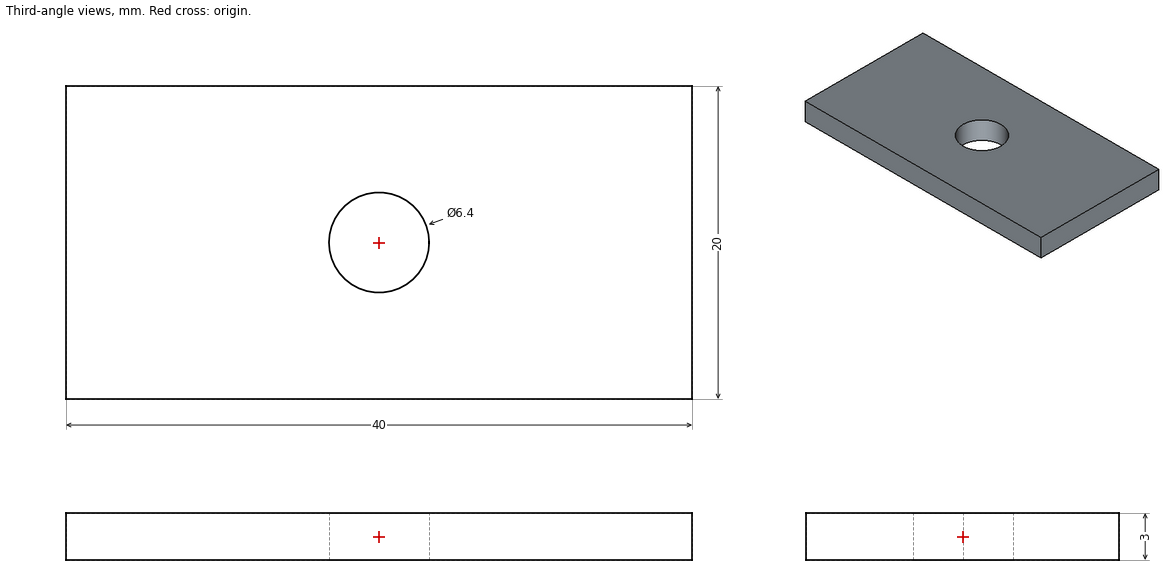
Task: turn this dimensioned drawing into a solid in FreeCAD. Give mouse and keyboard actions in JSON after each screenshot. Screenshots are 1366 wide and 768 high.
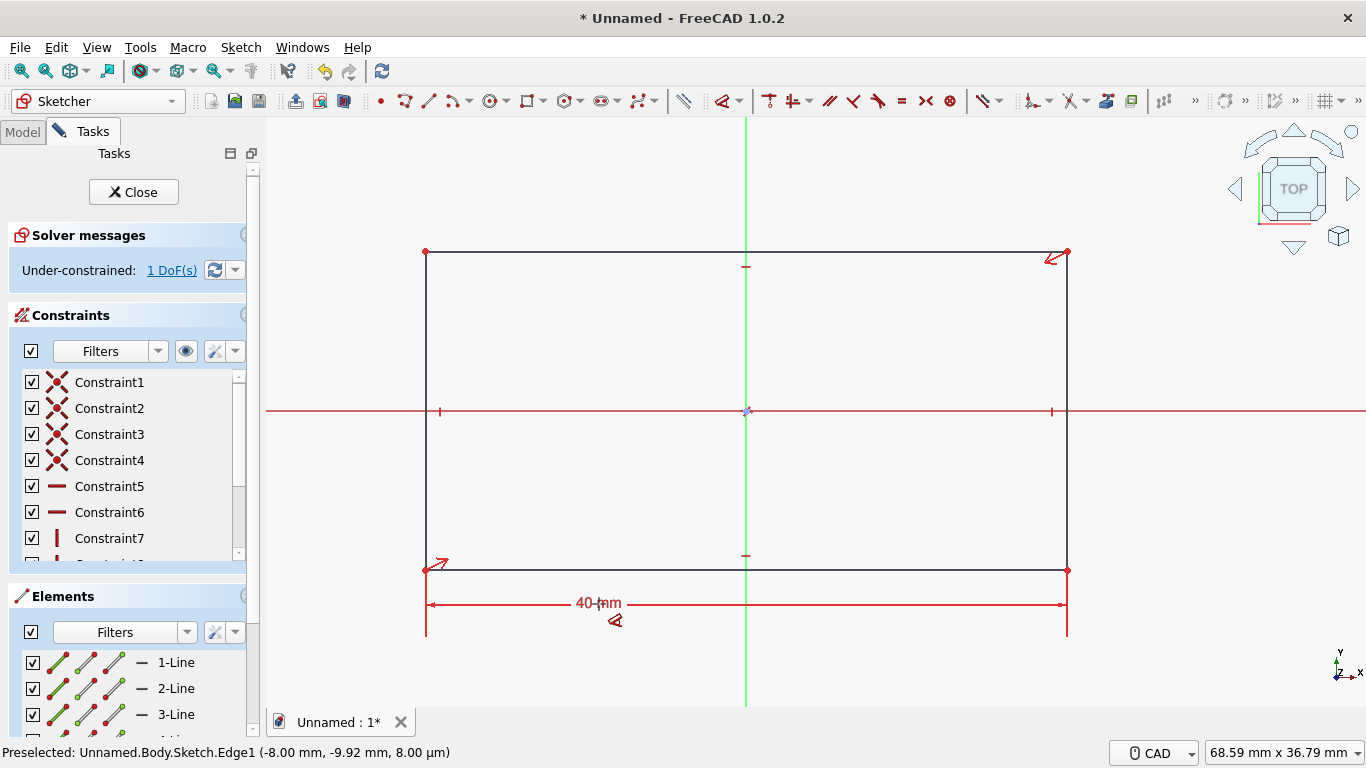
{"action": "left_click", "coordinate": [1067, 475]}
{"action": "left_click", "coordinate": [1101, 338]}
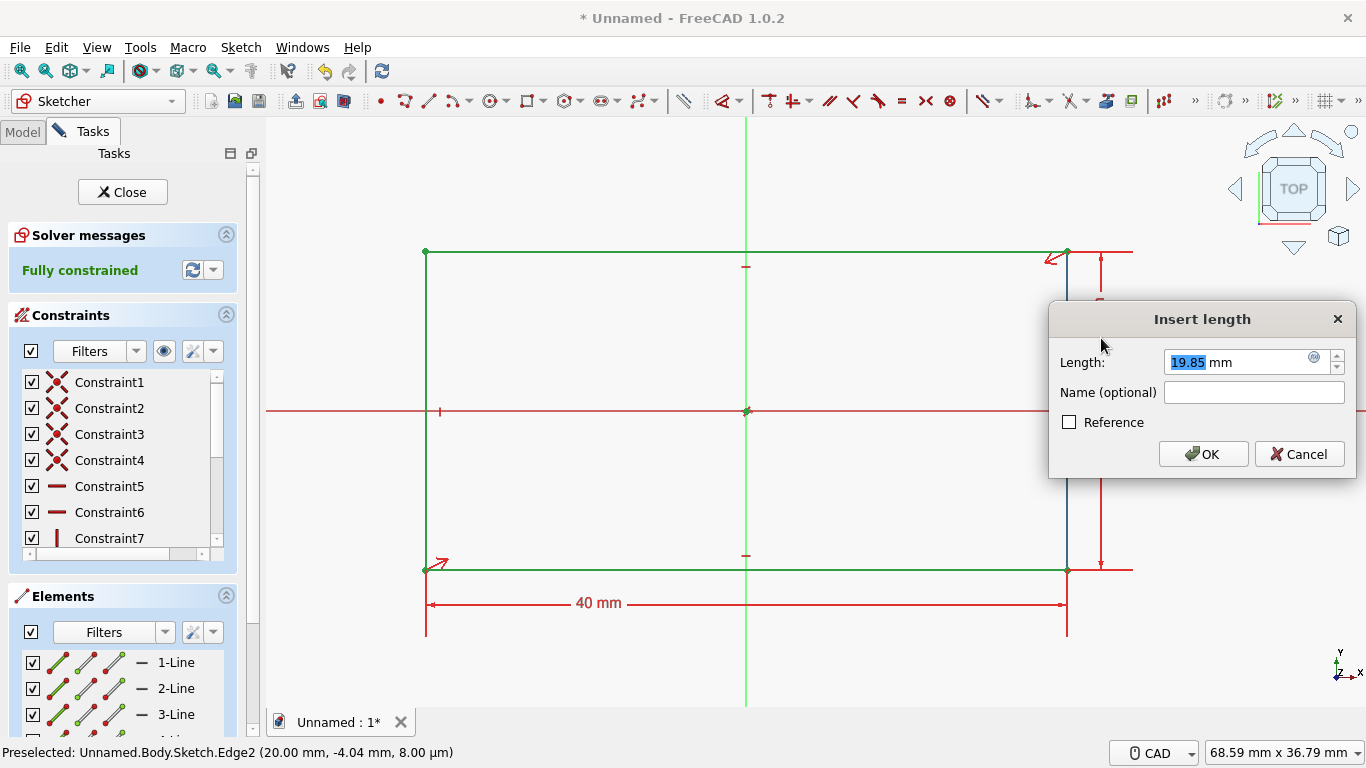
{"action": "type", "text": "20"}
{"action": "key", "text": "Return"}
{"action": "key", "text": "Escape"}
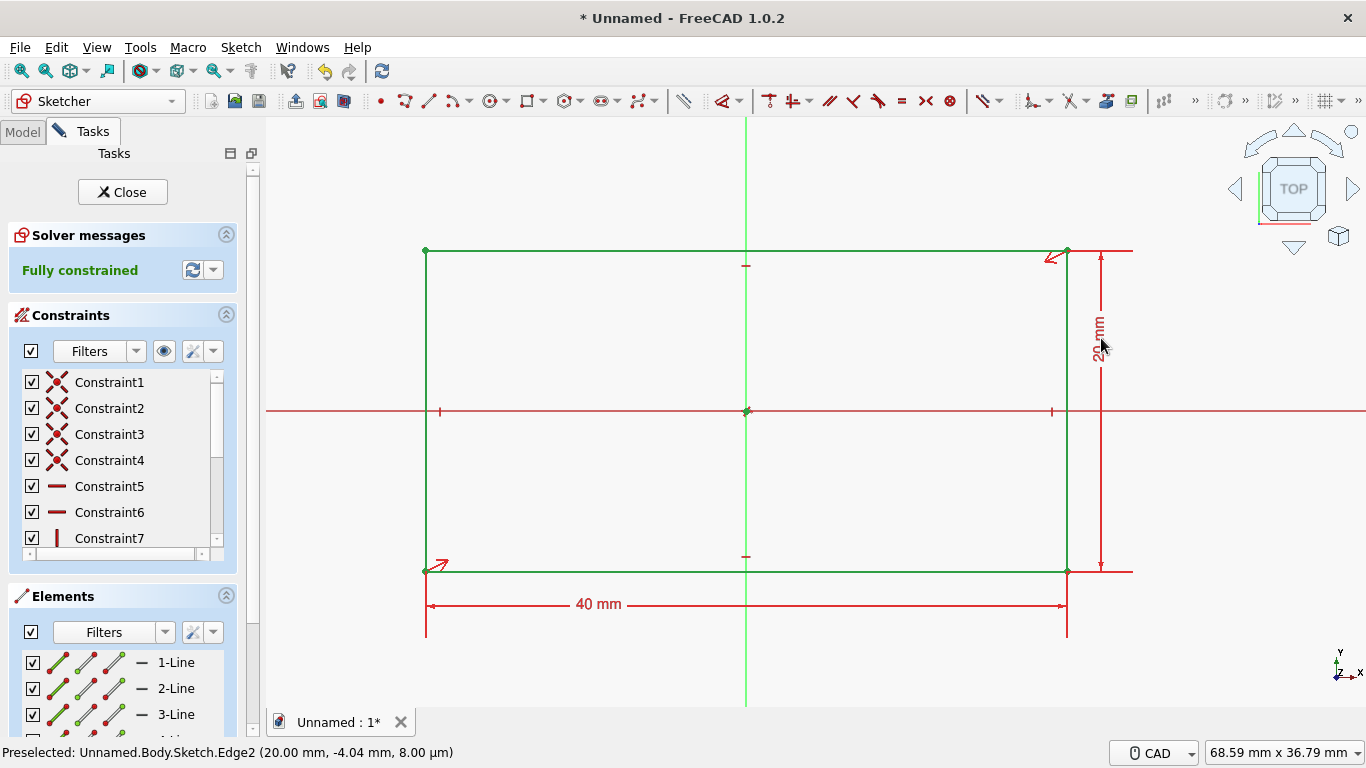
{"action": "left_click", "coordinate": [123, 192]}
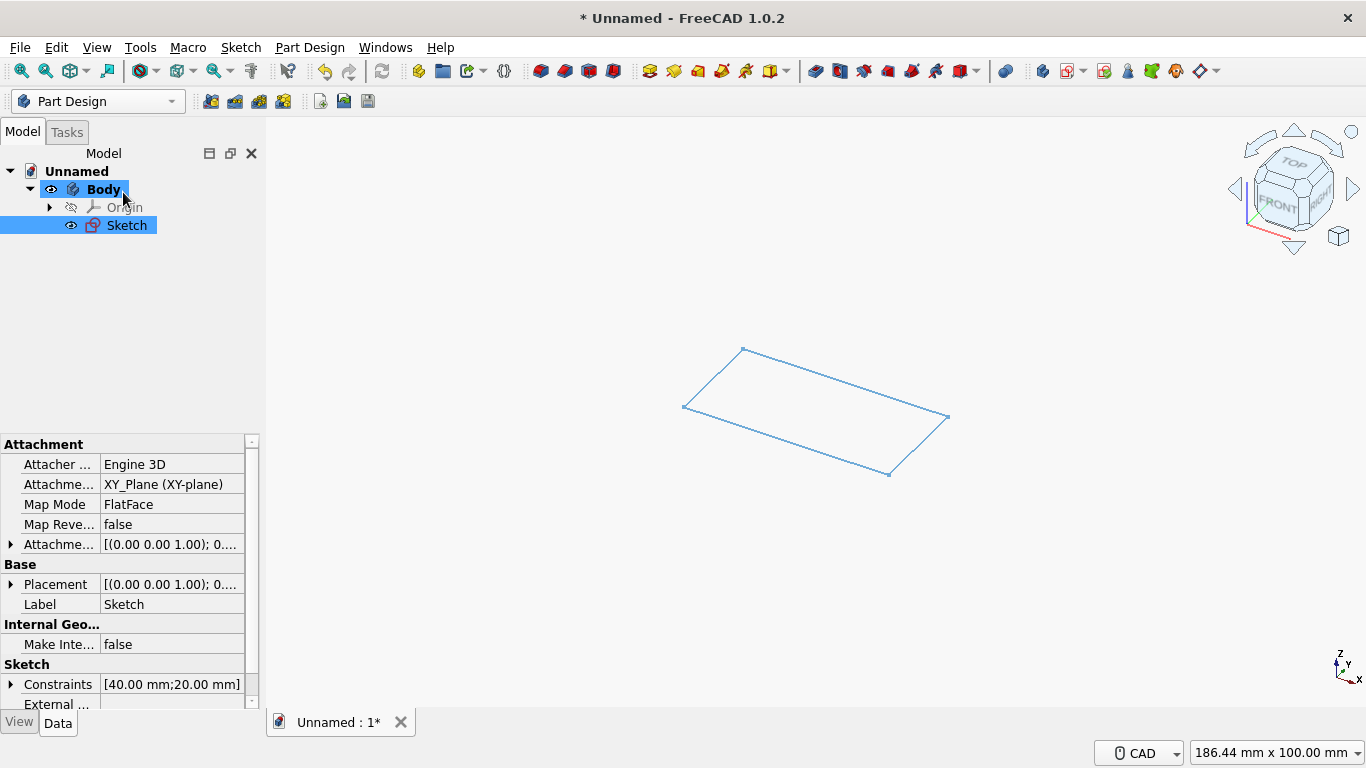
{"action": "left_click", "coordinate": [650, 72]}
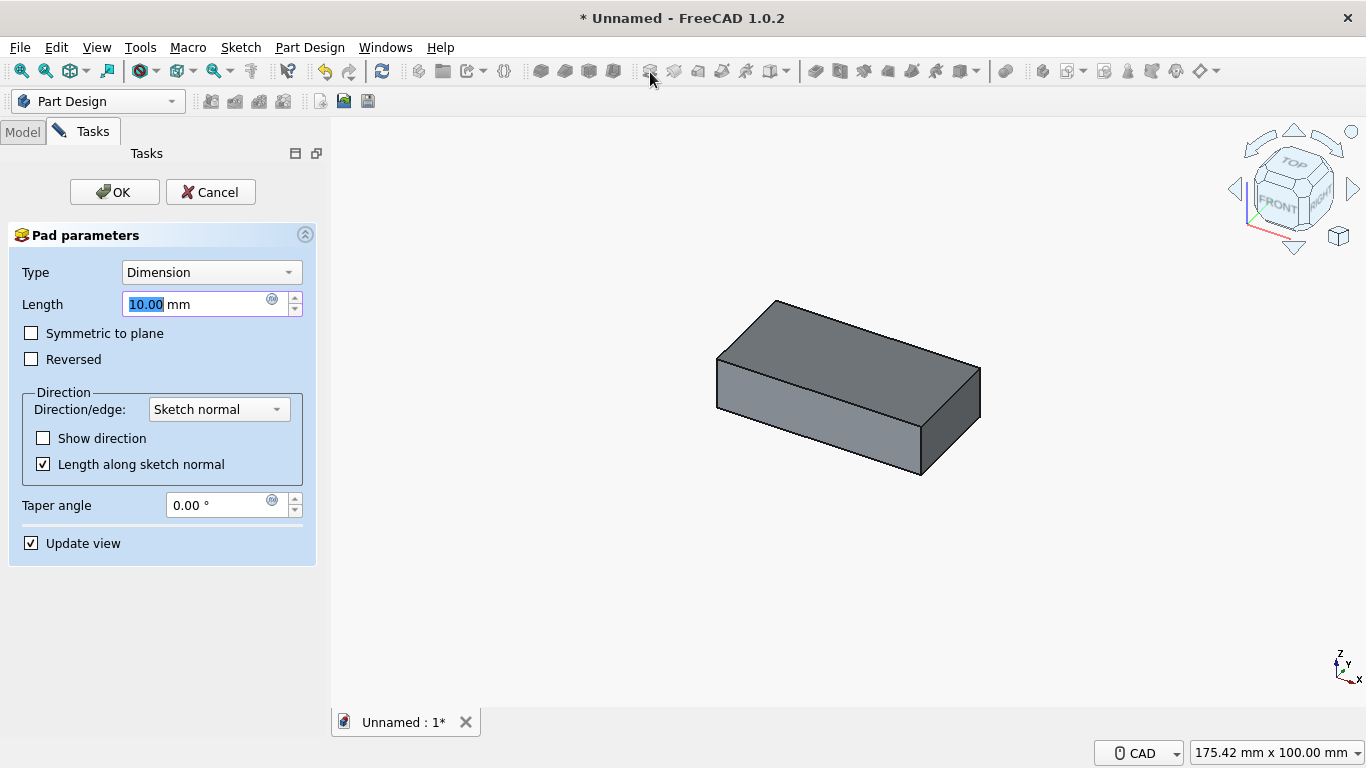
{"action": "type", "text": "3"}
{"action": "key", "text": "Tab"}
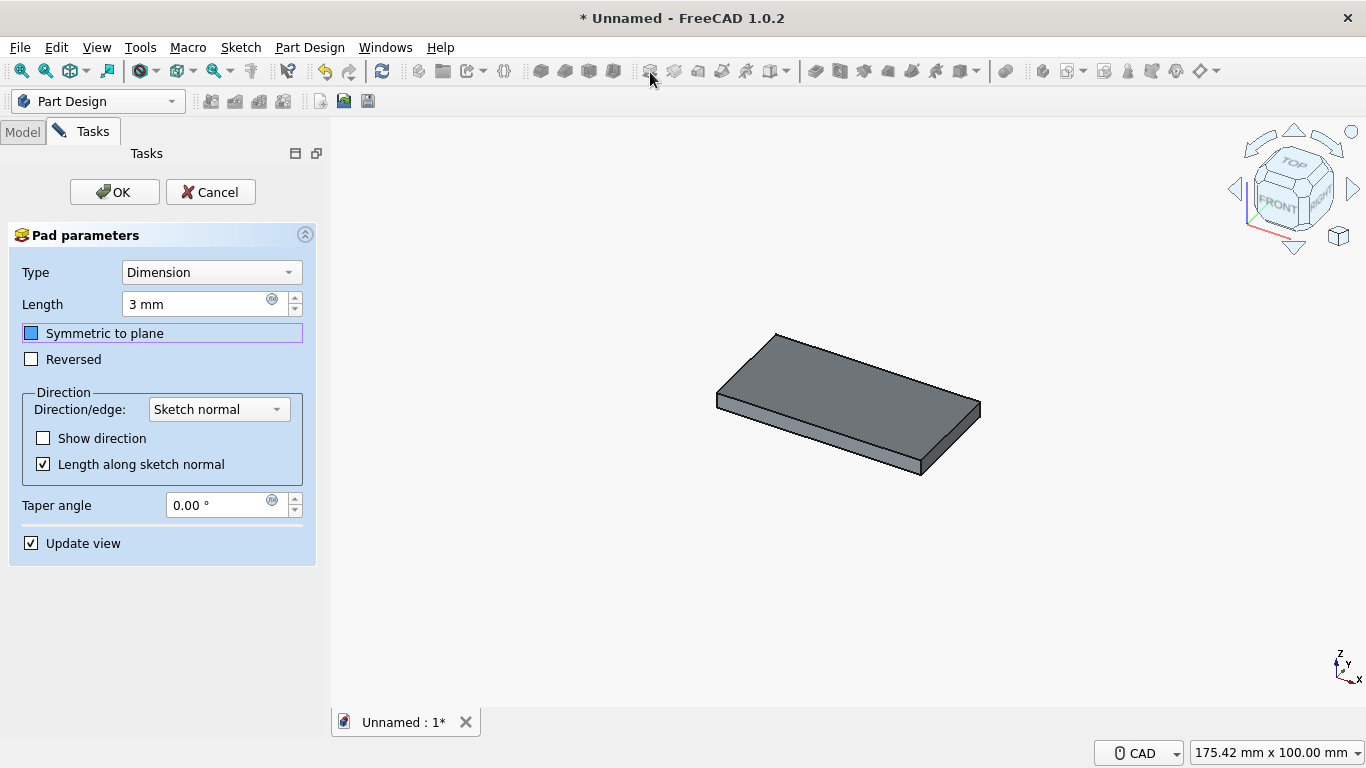
{"action": "left_click", "coordinate": [30, 333]}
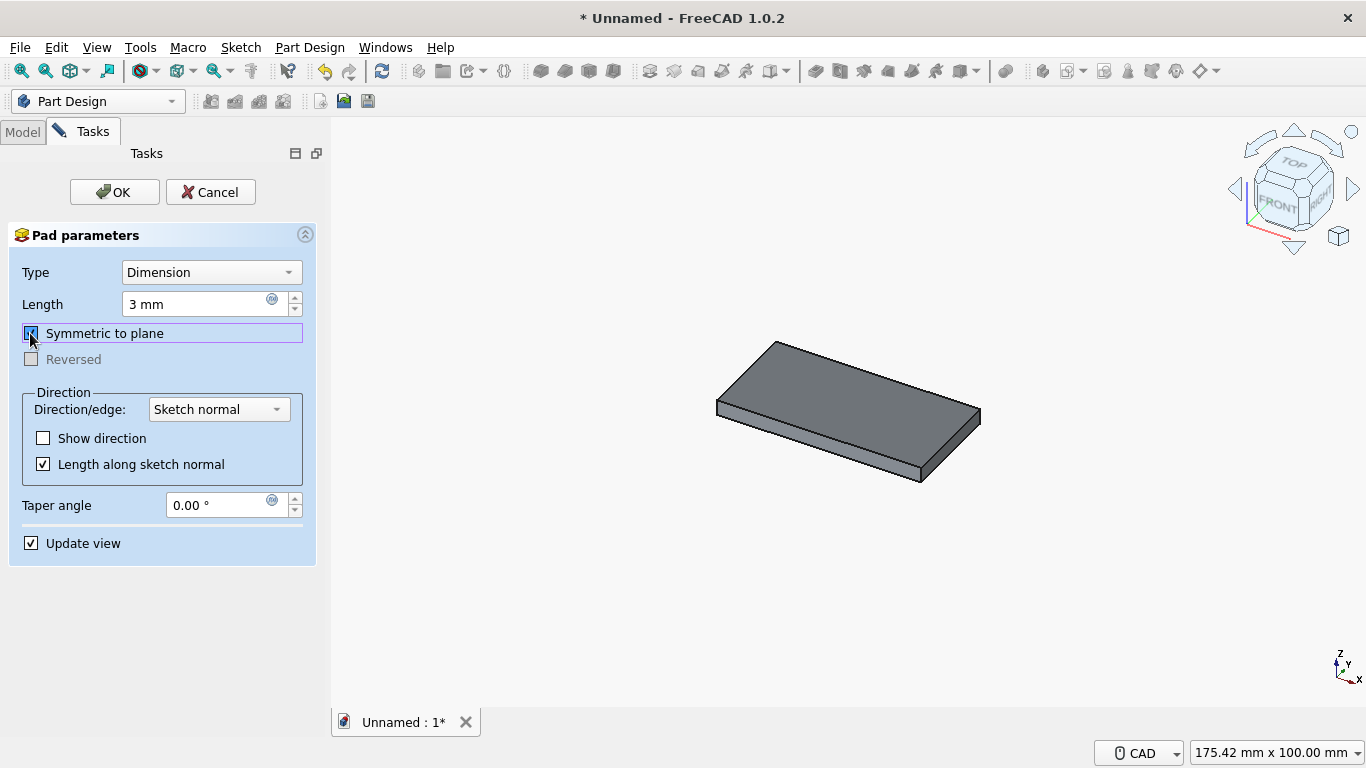
{"action": "left_click", "coordinate": [115, 192]}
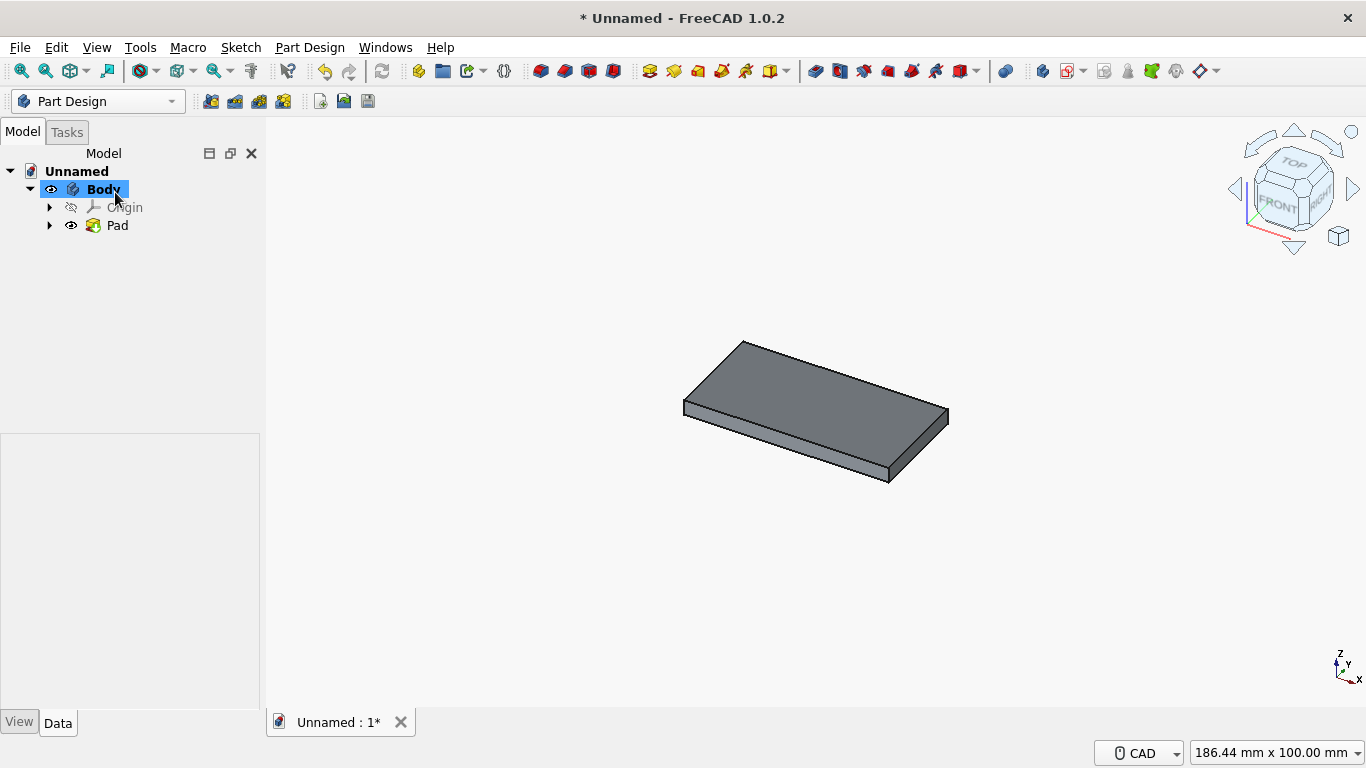
{"action": "key", "text": "v f"}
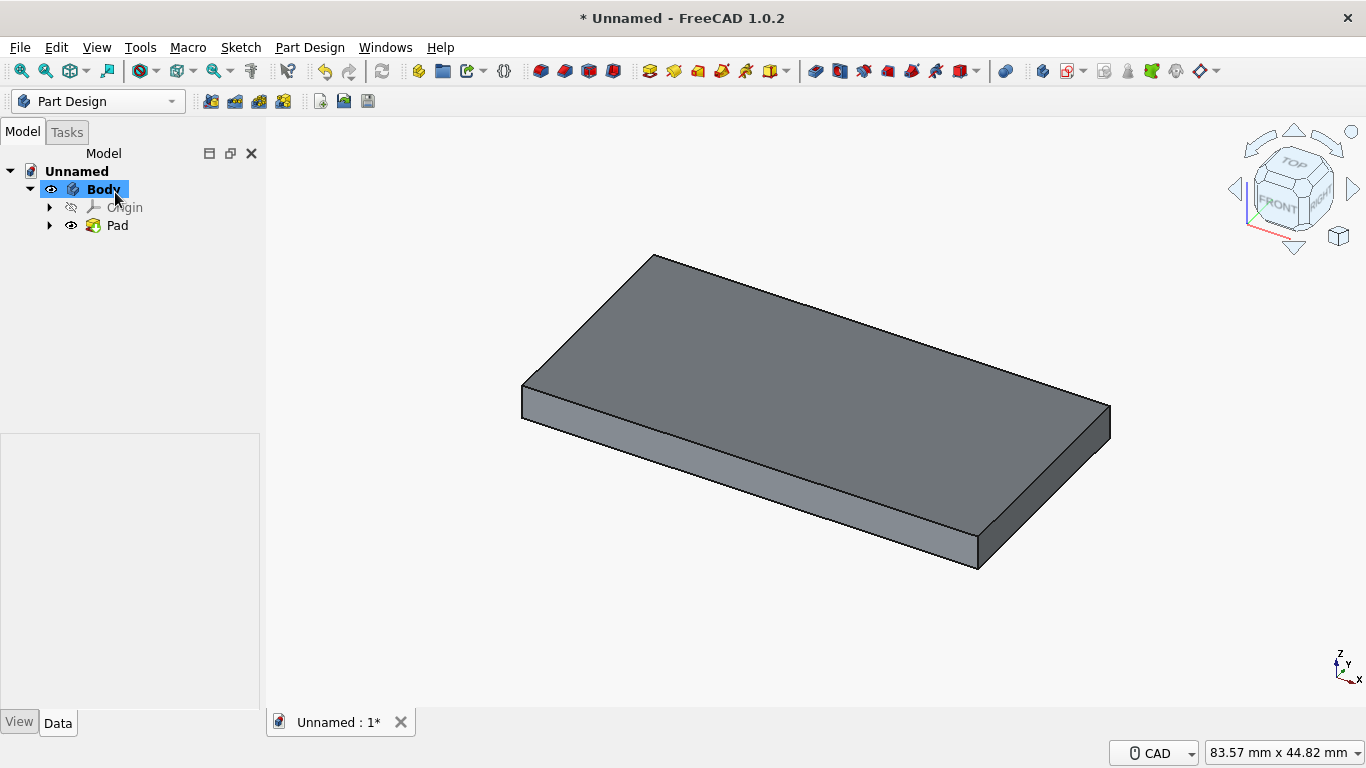
{"action": "left_click", "coordinate": [1068, 72]}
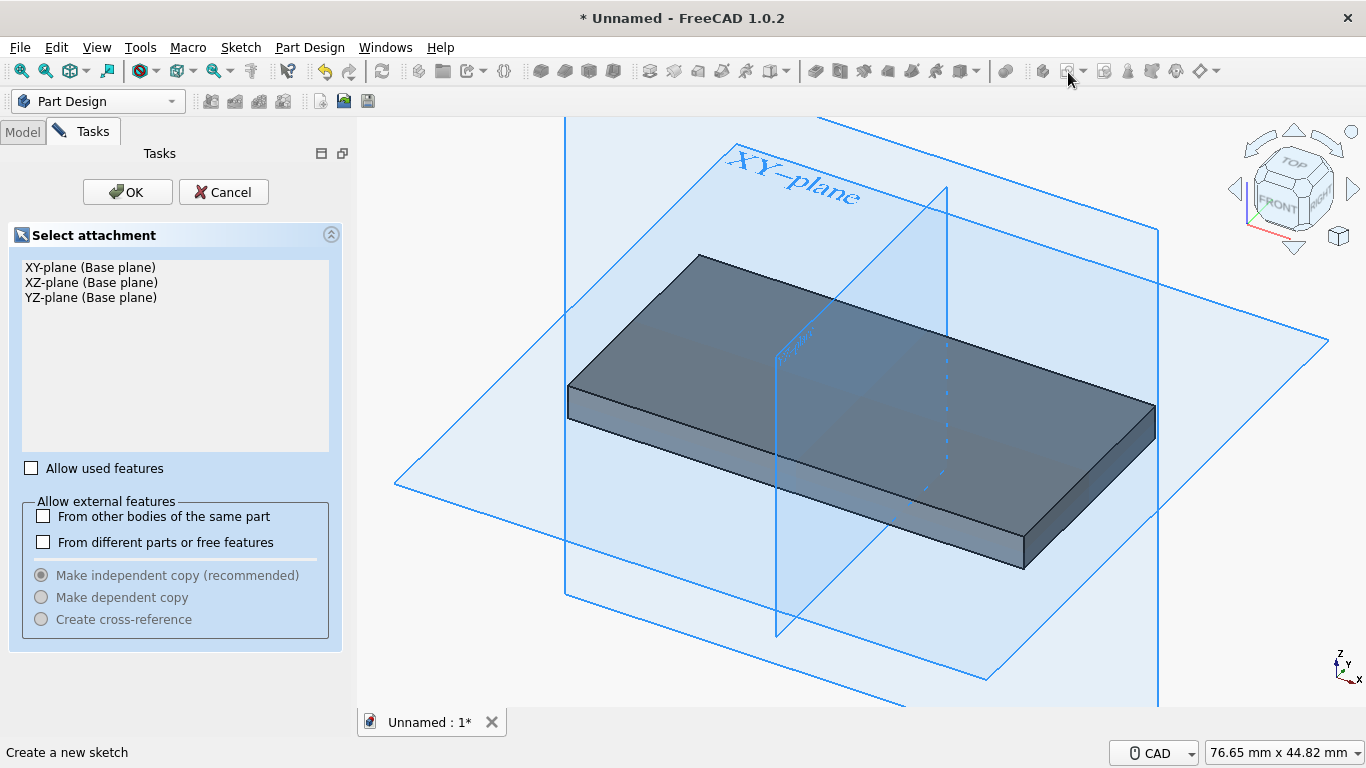
{"action": "left_click", "coordinate": [82, 268]}